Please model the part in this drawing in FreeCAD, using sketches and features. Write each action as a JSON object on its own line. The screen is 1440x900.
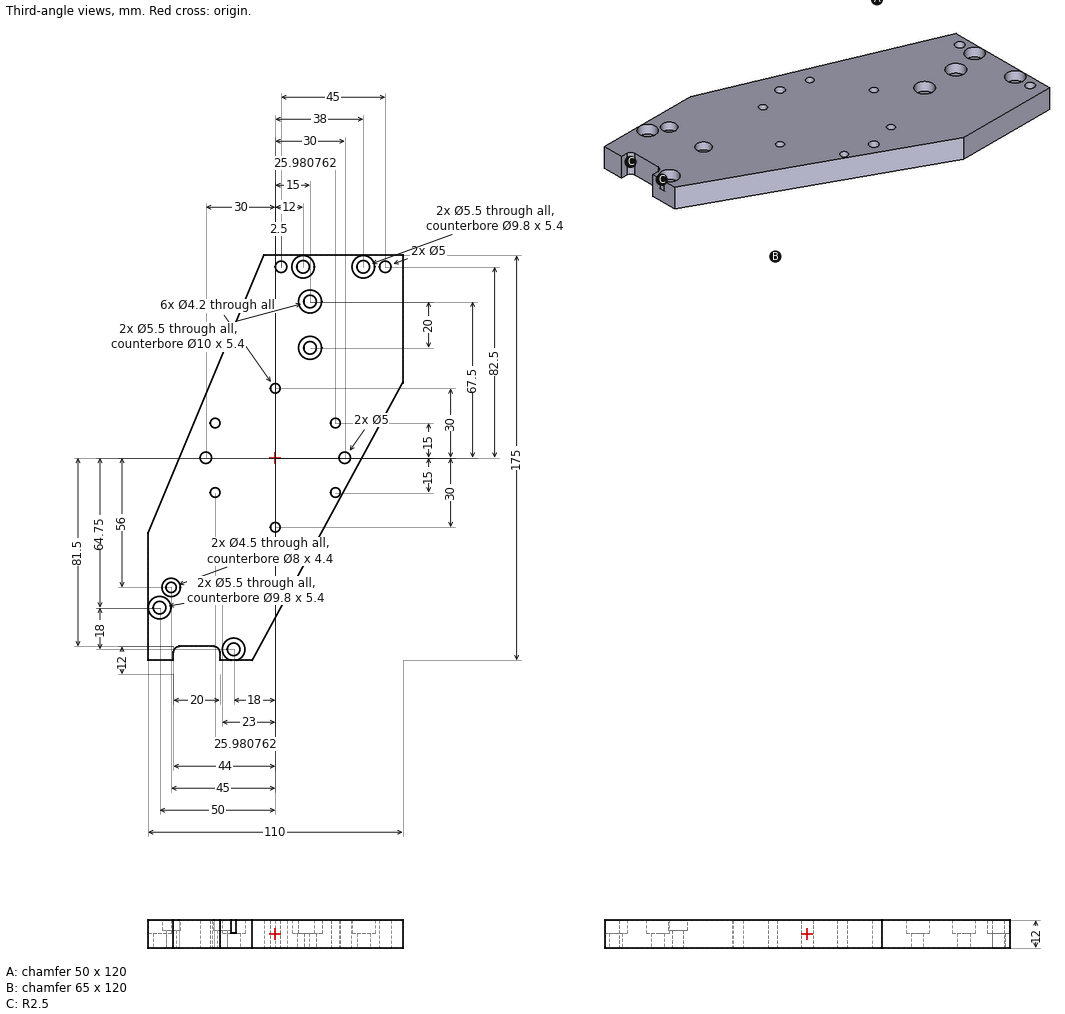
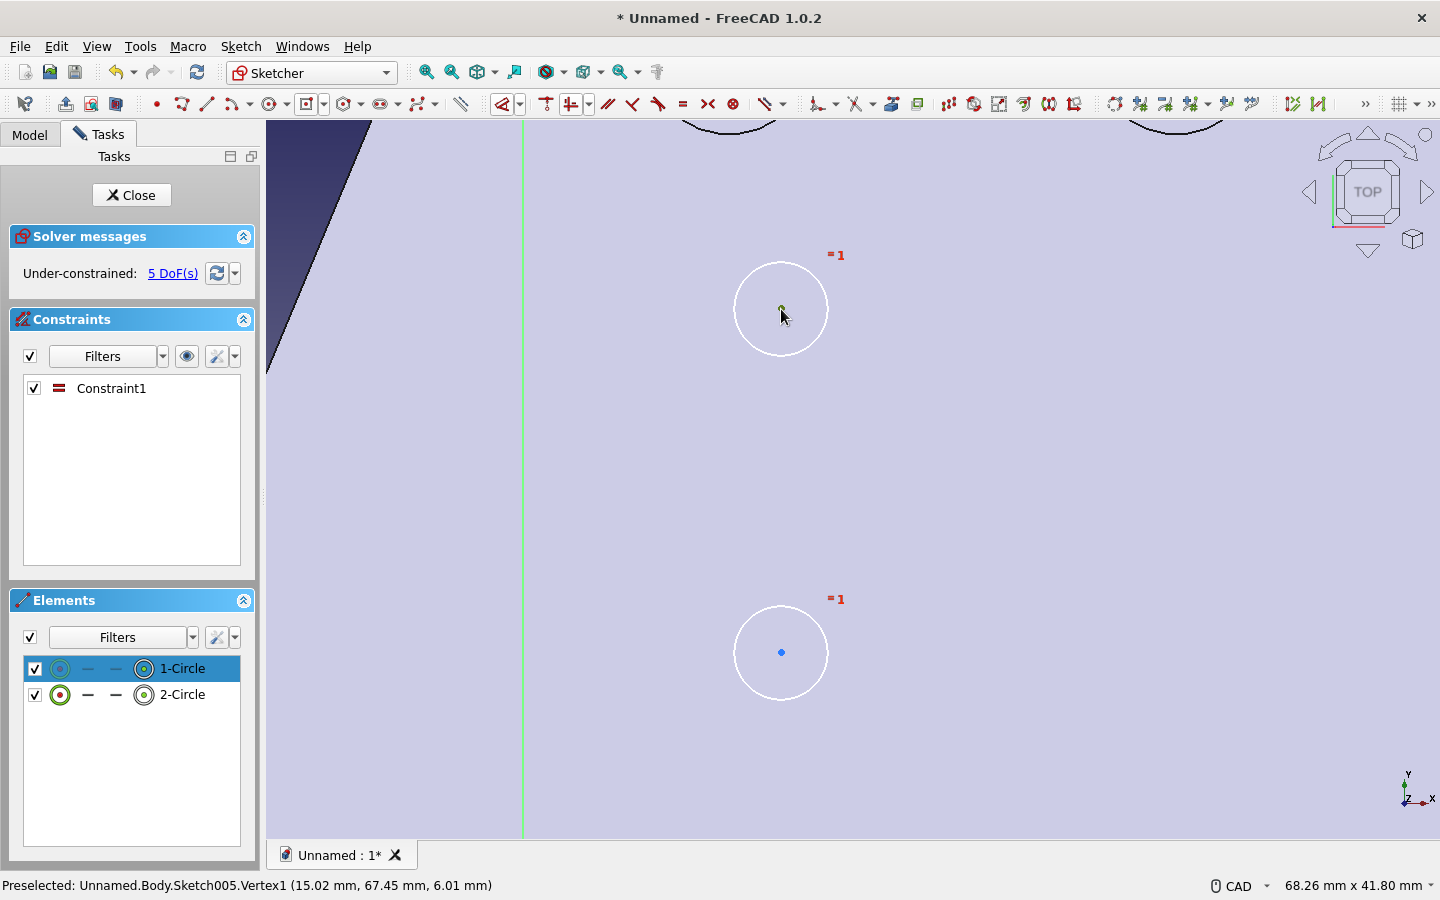
{"action": "left_click", "coordinate": [781, 653]}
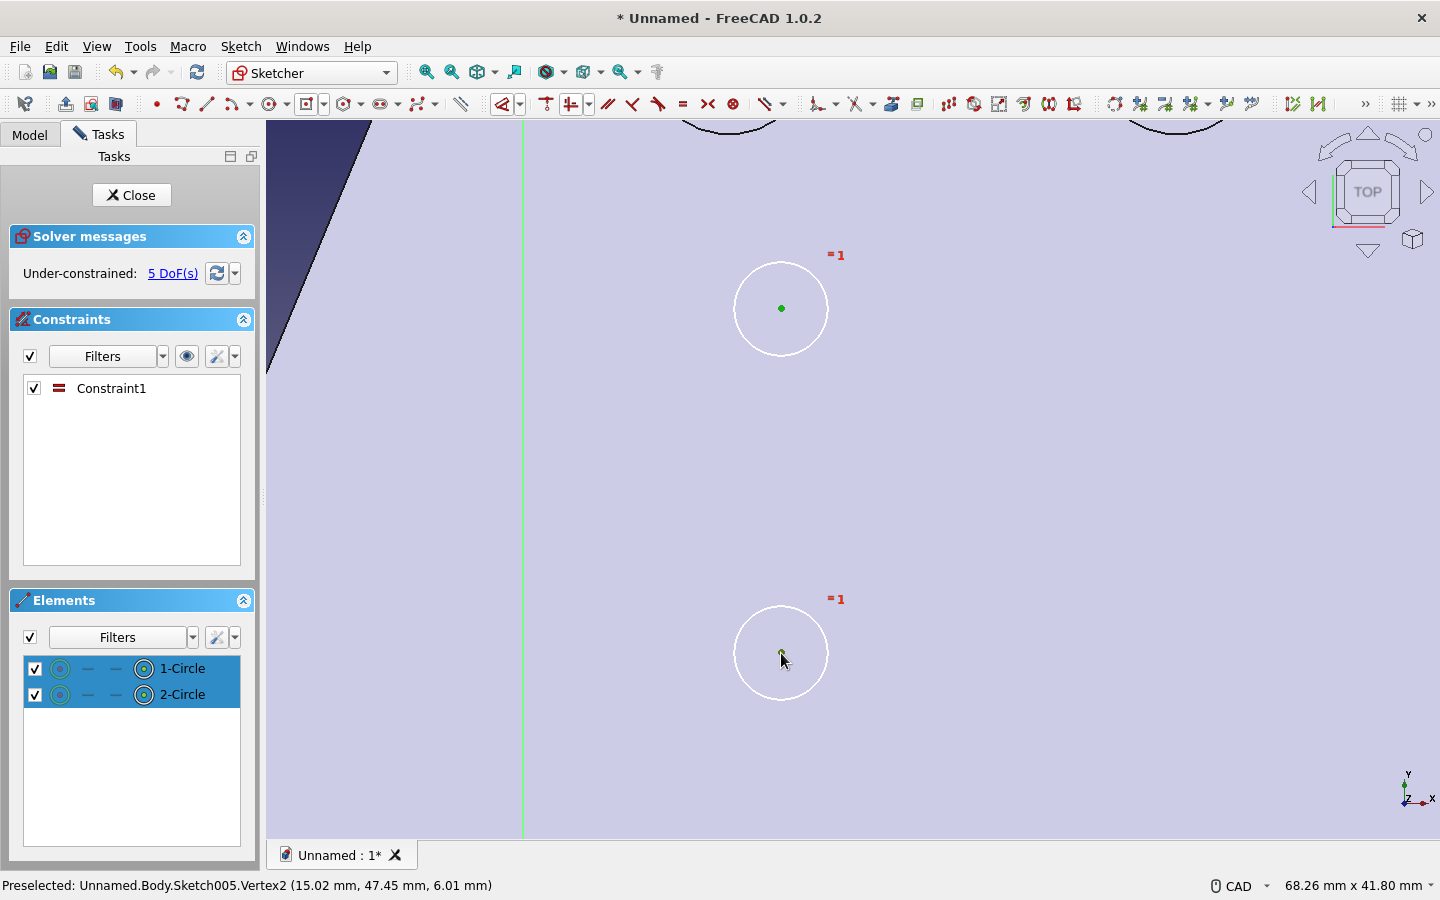
{"action": "key", "text": "v"}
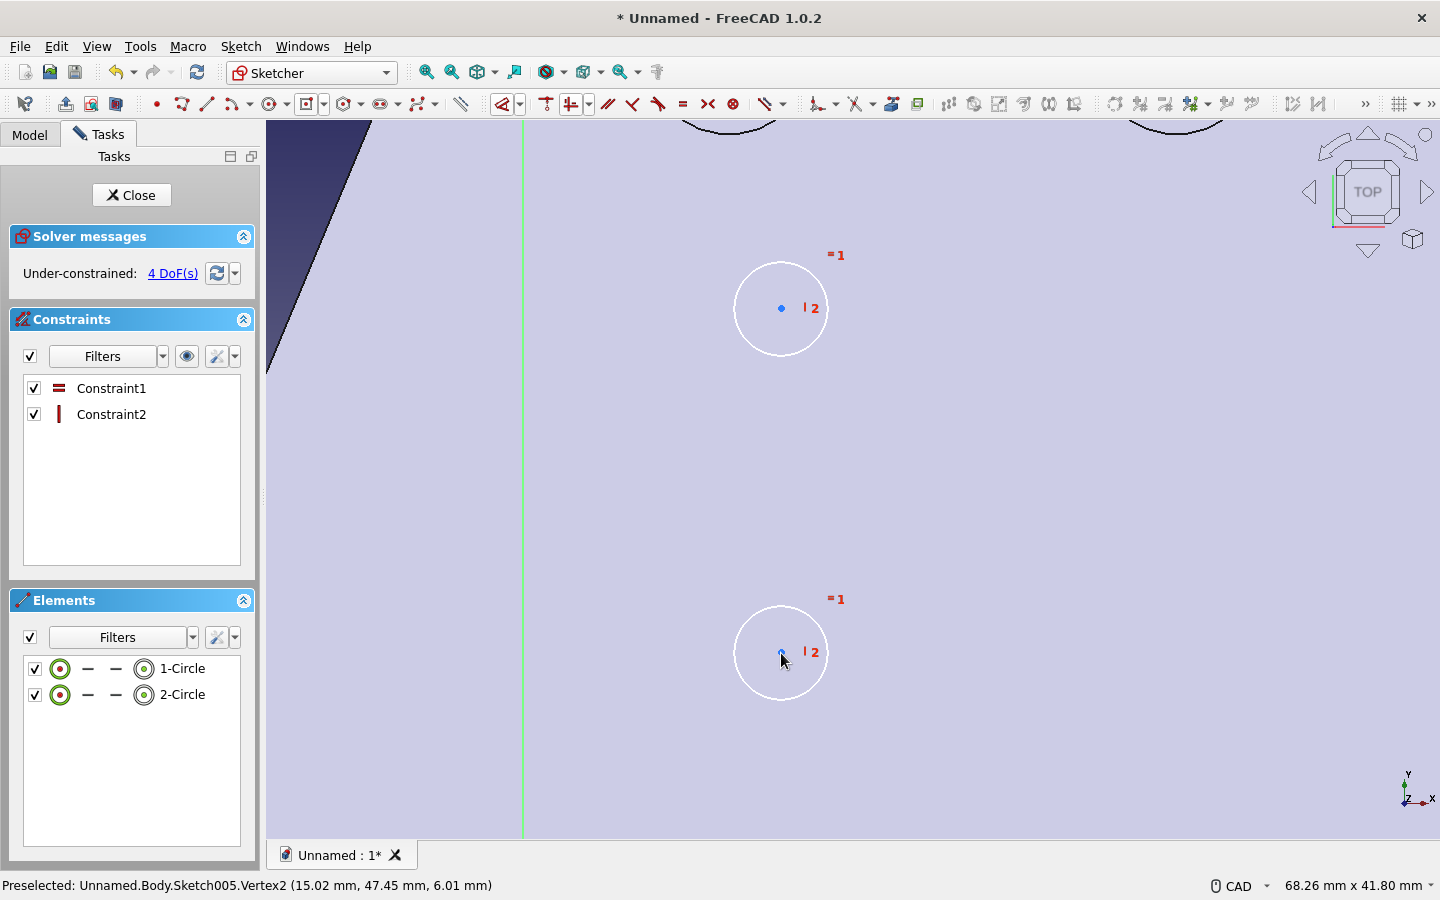
{"action": "left_click", "coordinate": [814, 276]}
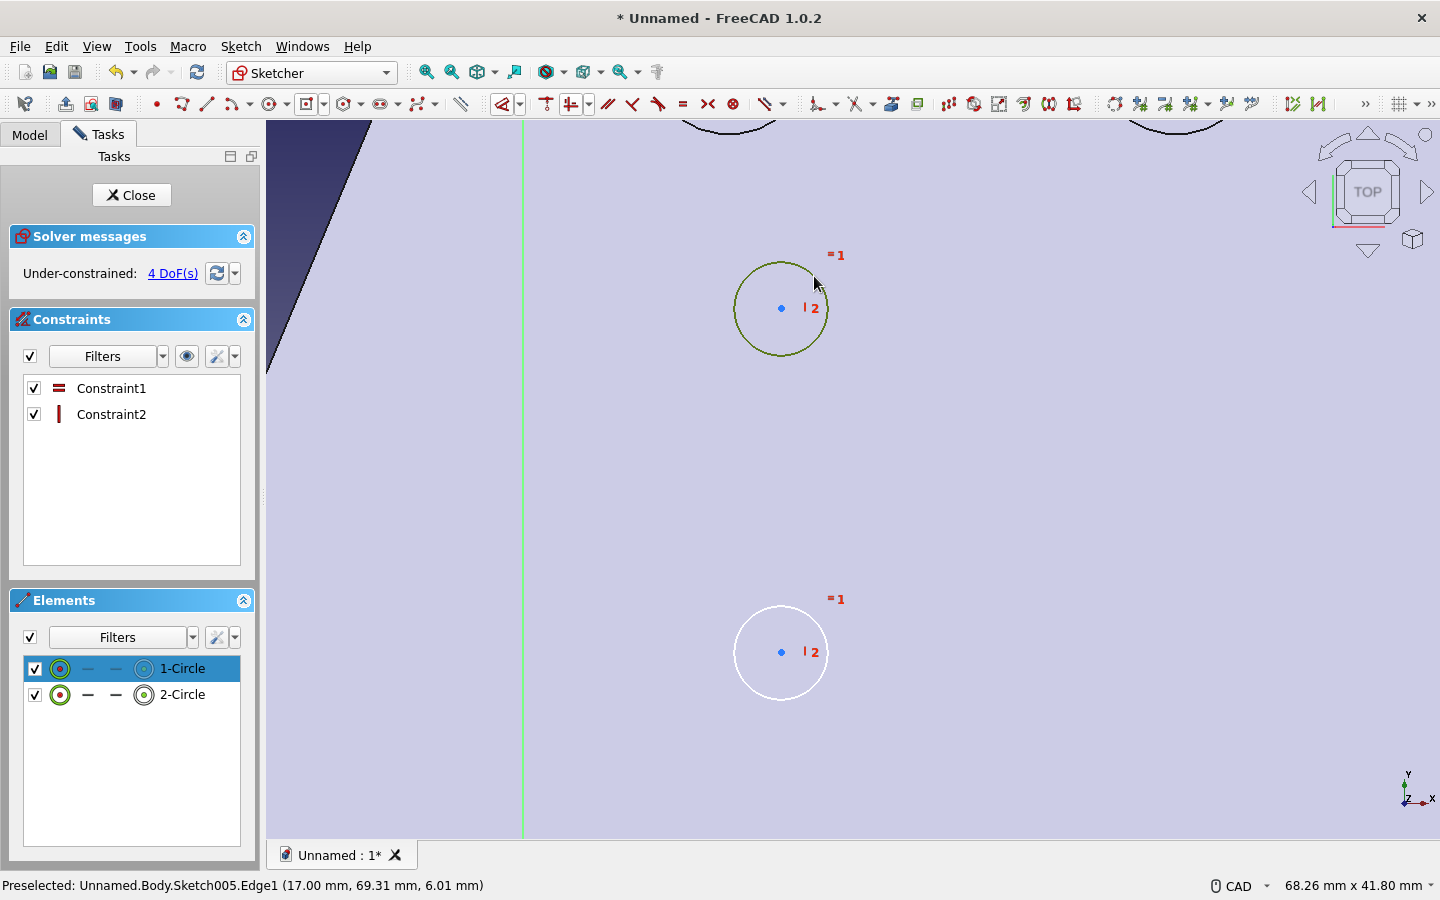
{"action": "key", "text": "k o"}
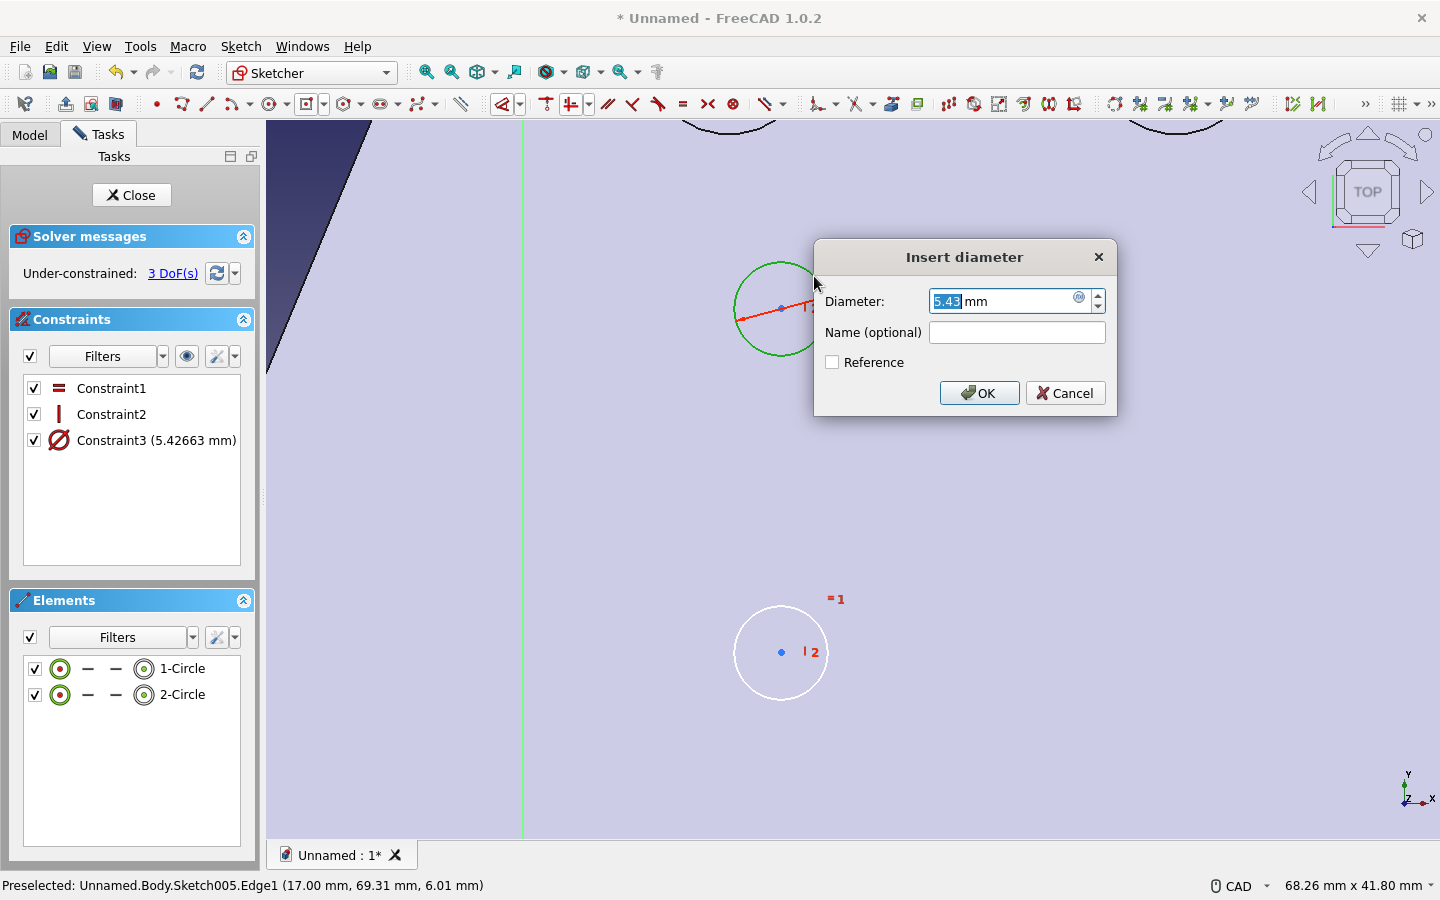
{"action": "type", "text": "5.5"}
{"action": "key", "text": "Return"}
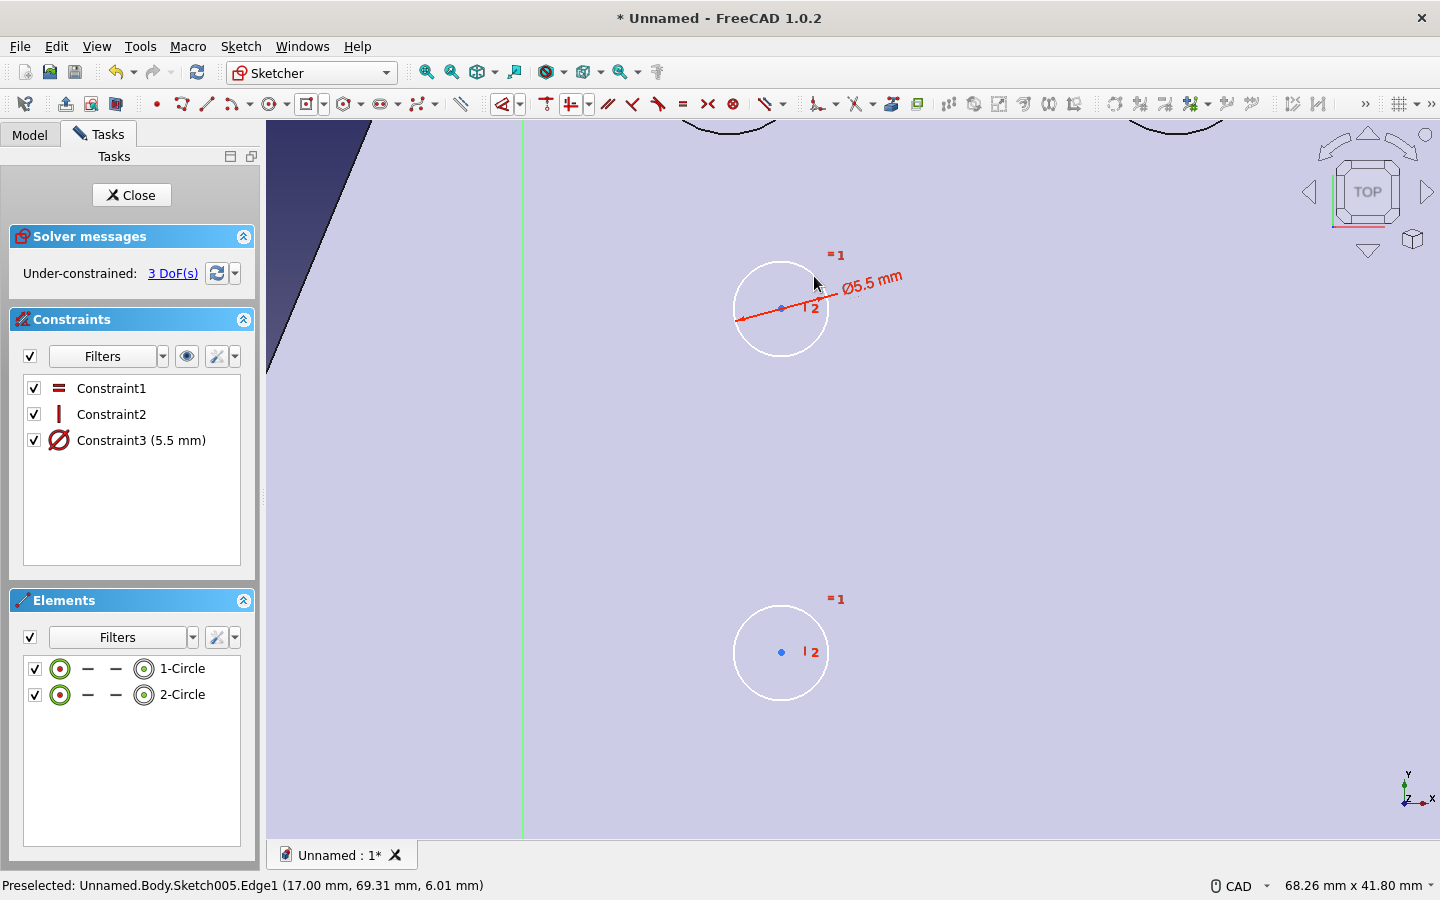
{"action": "left_click", "coordinate": [781, 309]}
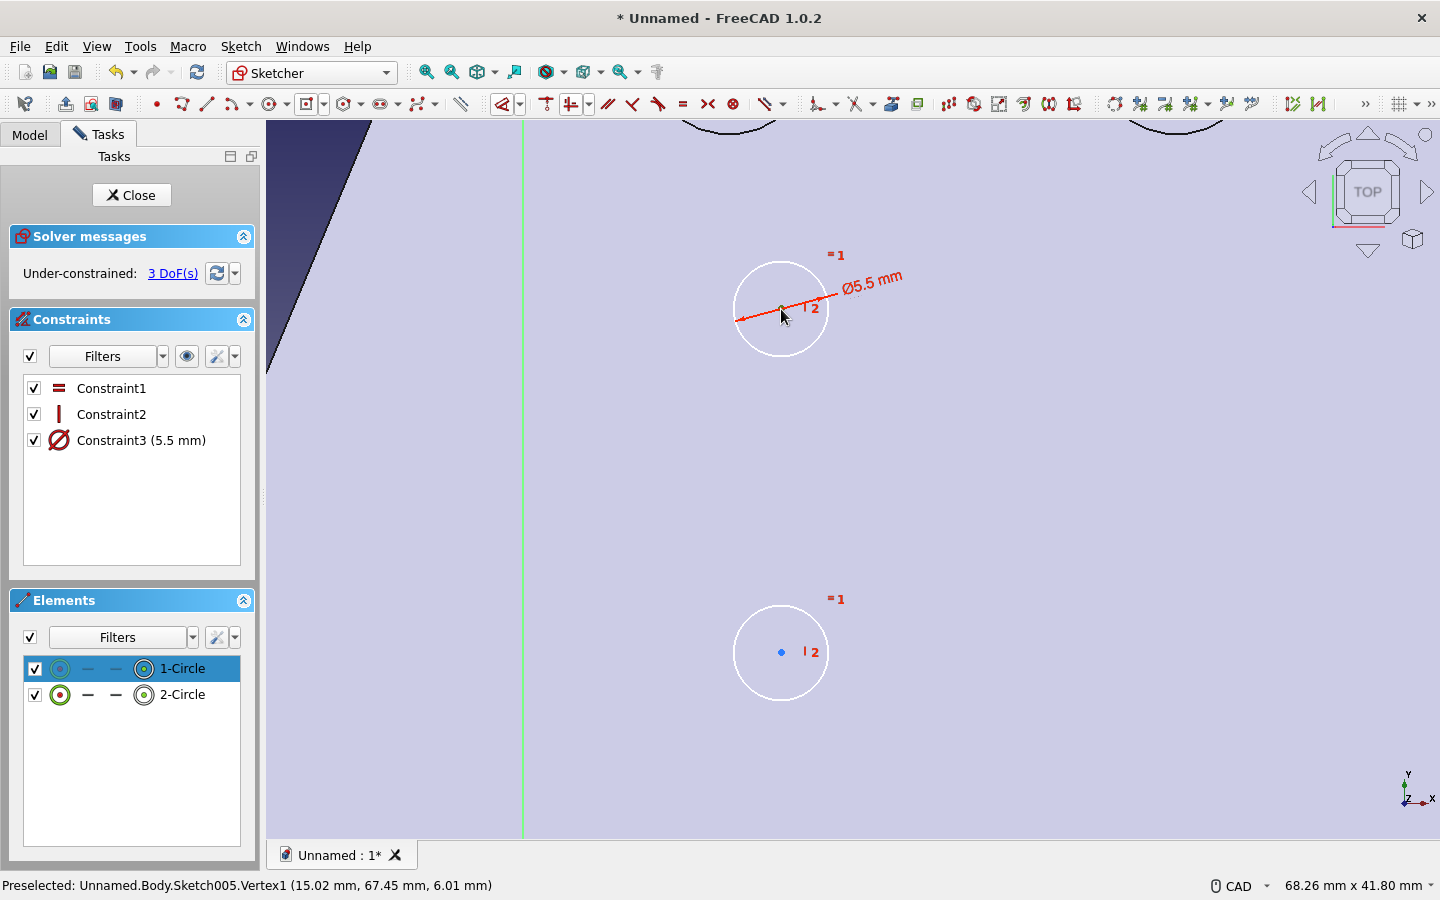
{"action": "left_click", "coordinate": [520, 104]}